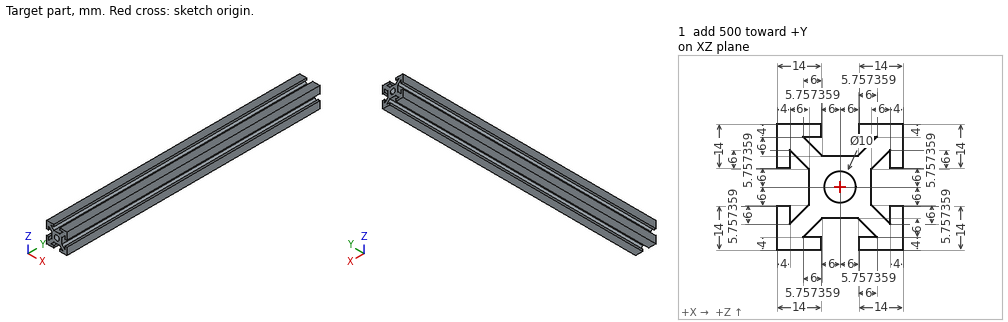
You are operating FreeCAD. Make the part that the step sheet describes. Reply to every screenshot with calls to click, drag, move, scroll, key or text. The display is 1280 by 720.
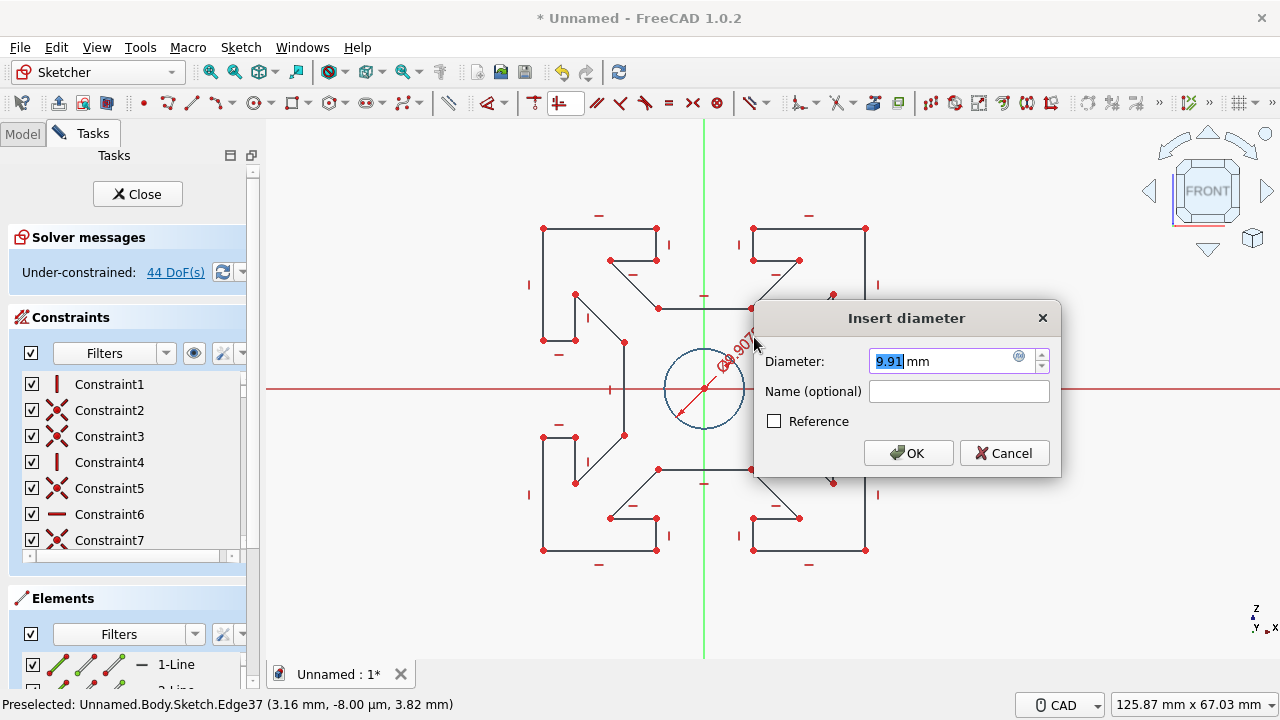
text(10)
key(Return)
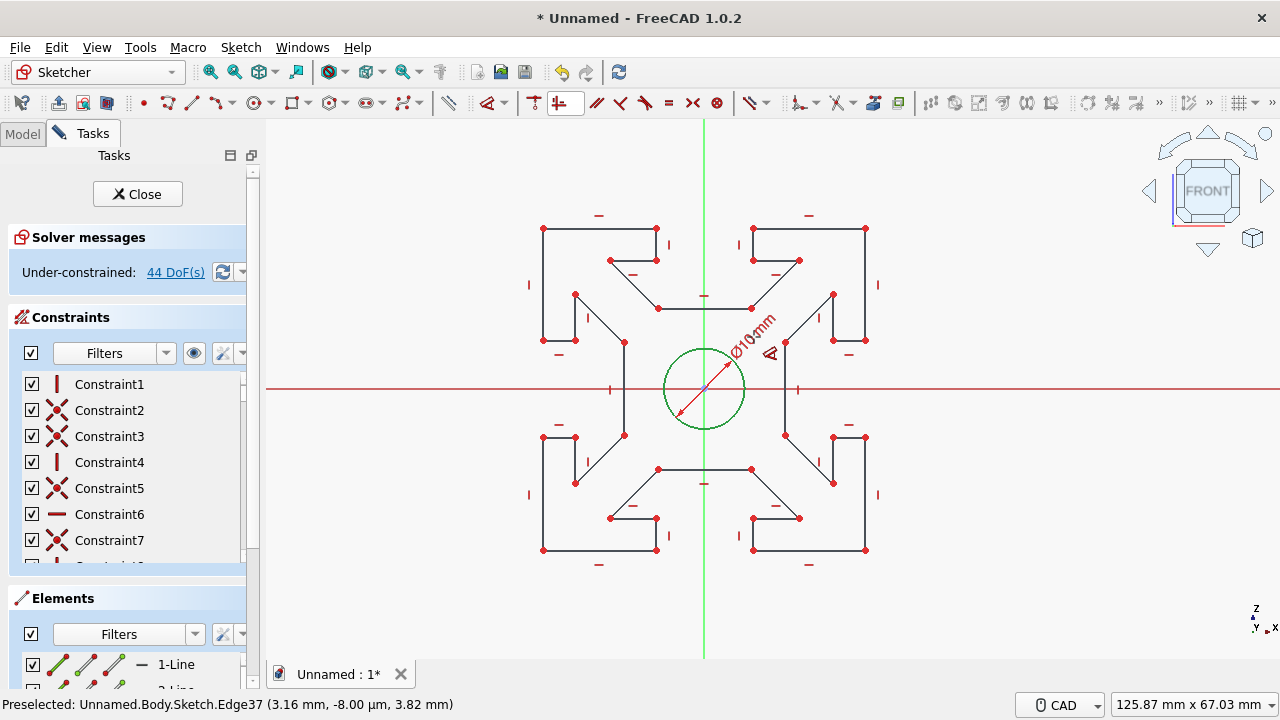
scroll(565, 341, up, 2)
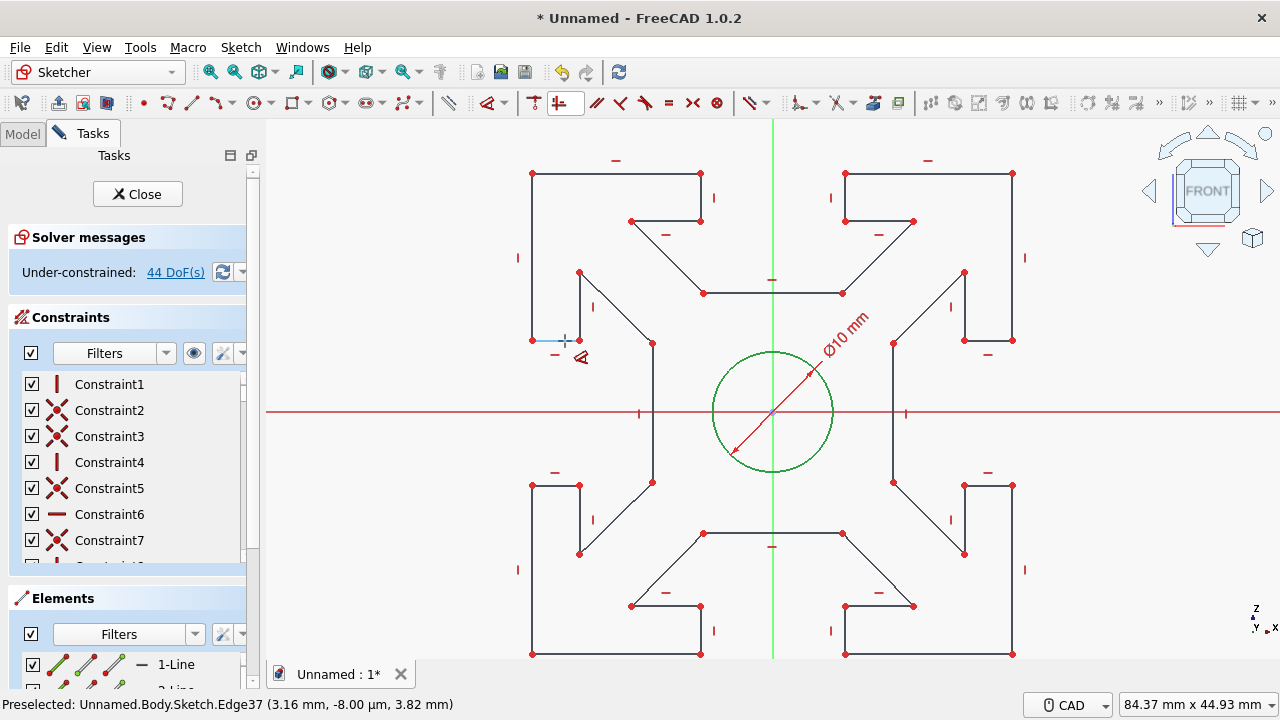
click(565, 341)
click(556, 307)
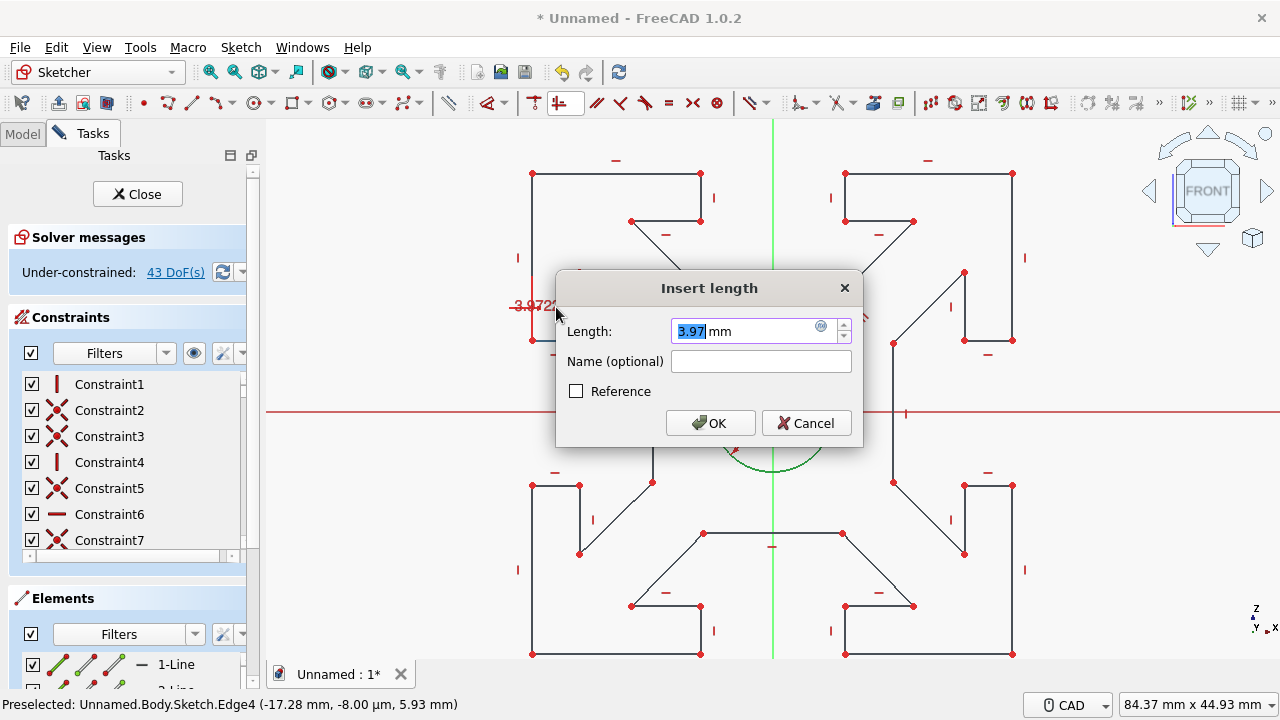
text(4)
key(Return)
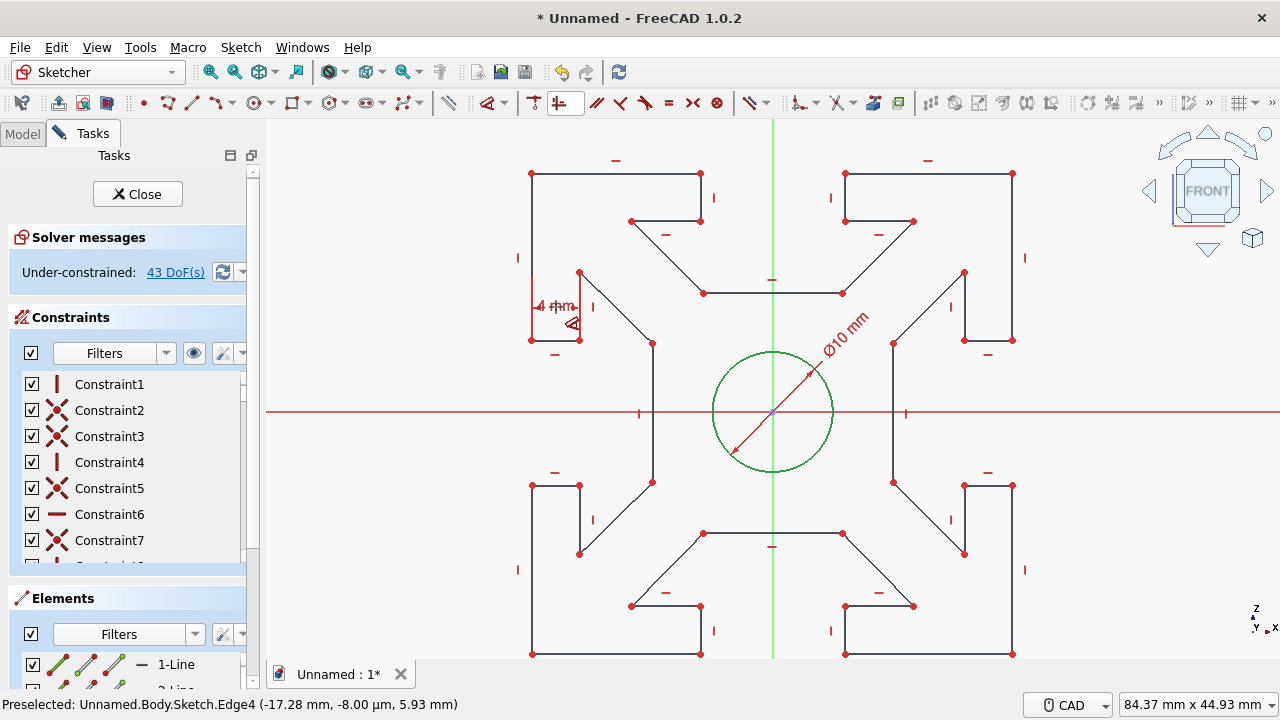
click(701, 188)
click(667, 198)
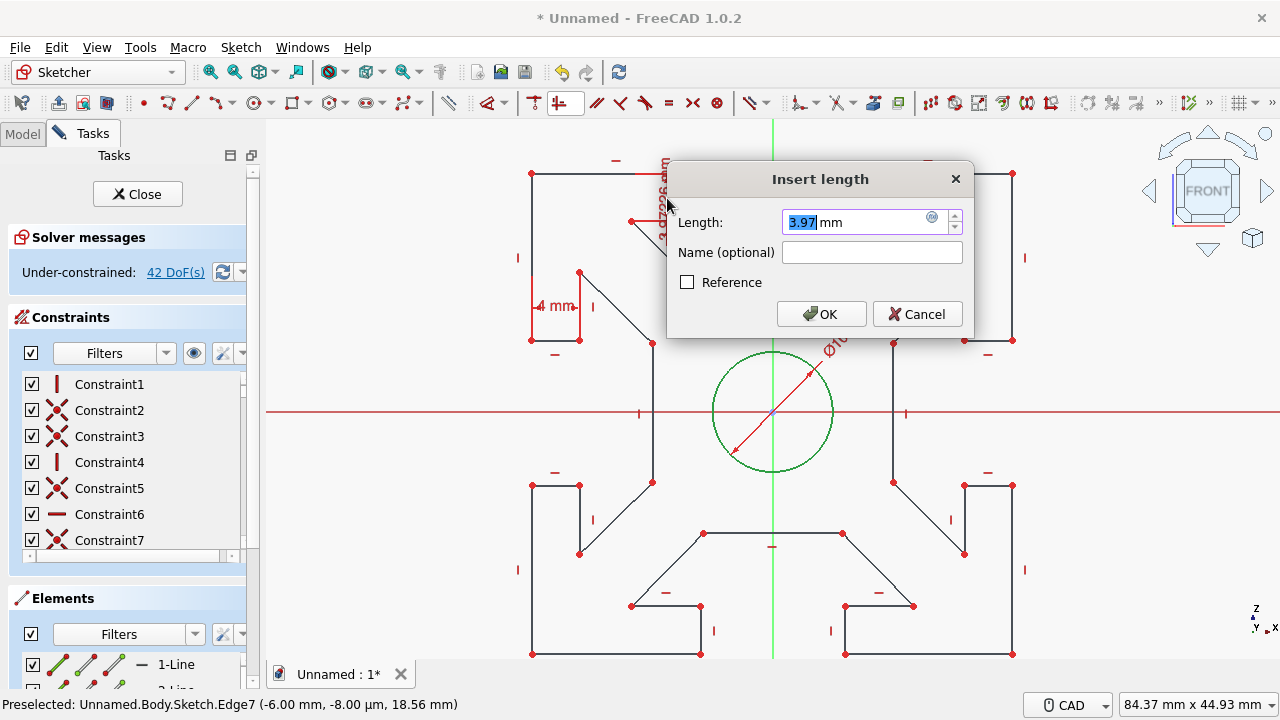
text(4)
key(Return)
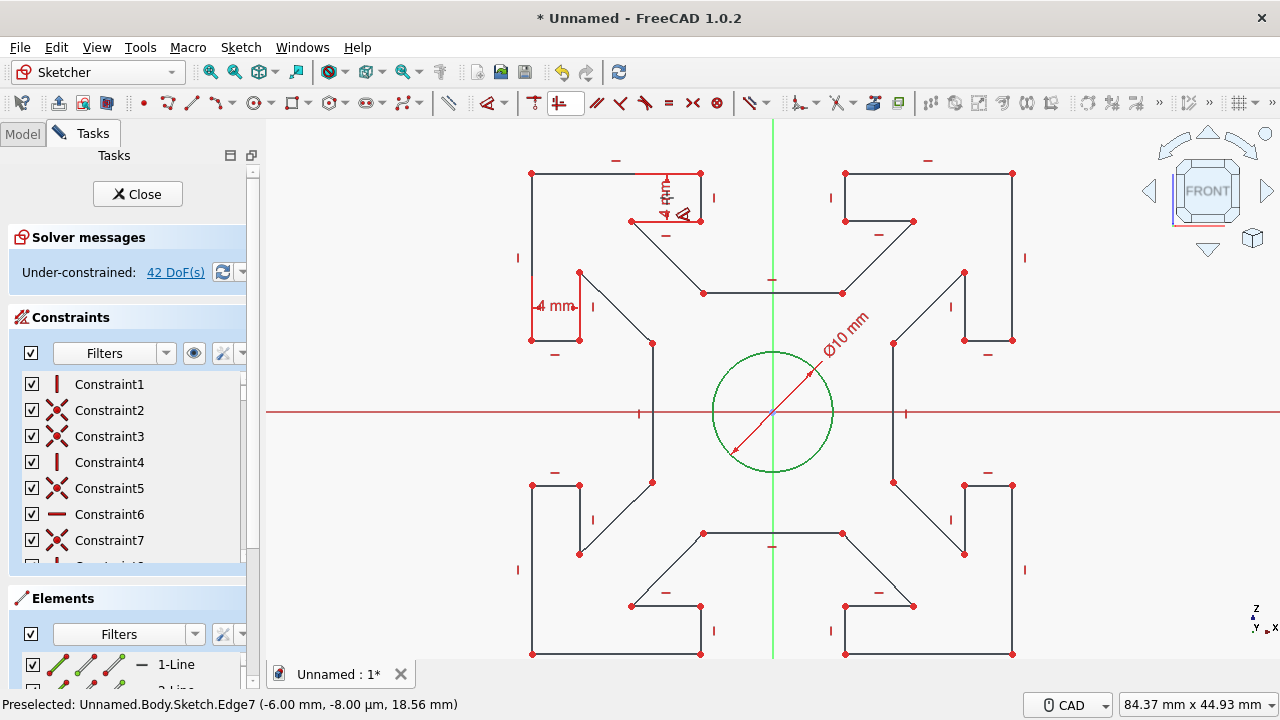
click(845, 207)
click(879, 198)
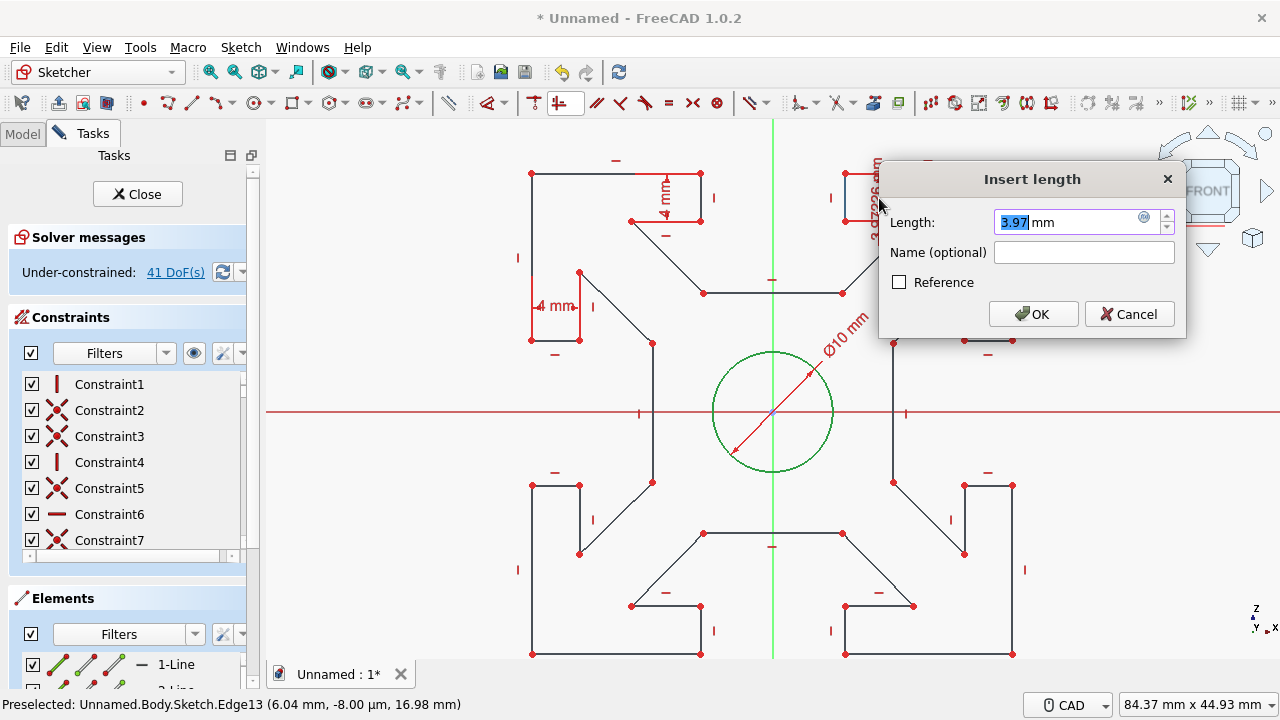
text(4)
key(Return)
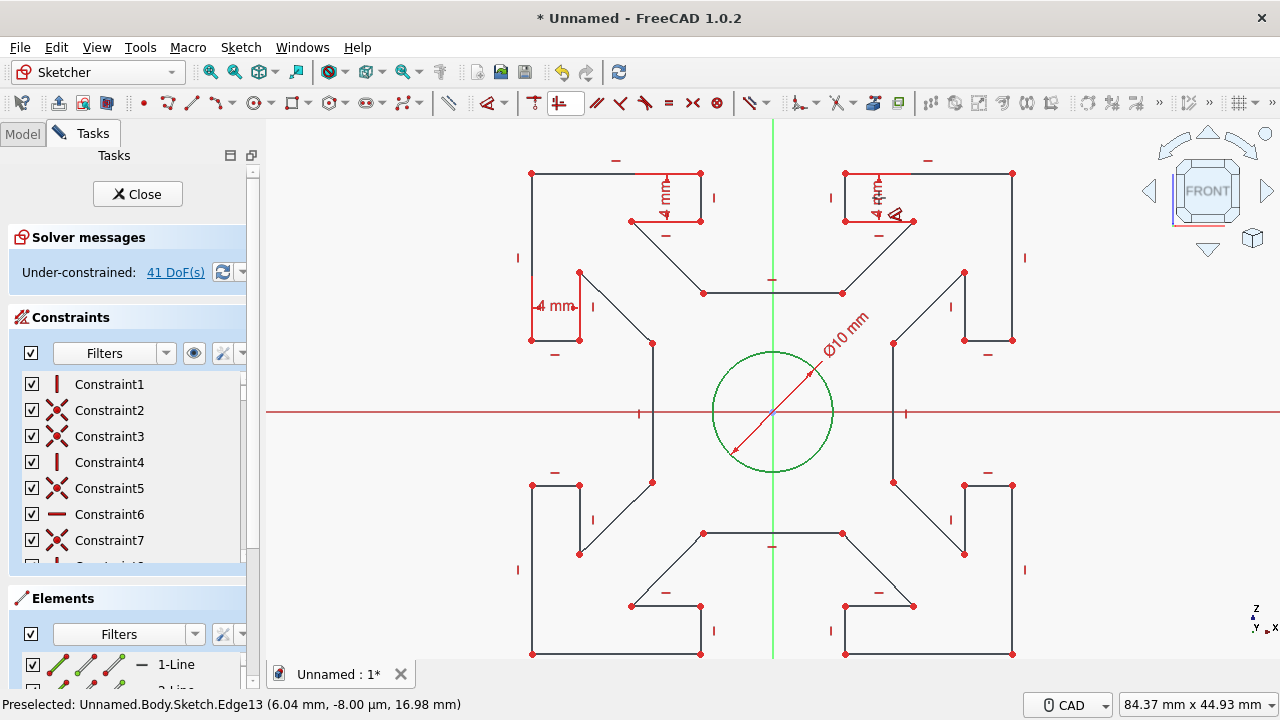
click(998, 341)
click(989, 307)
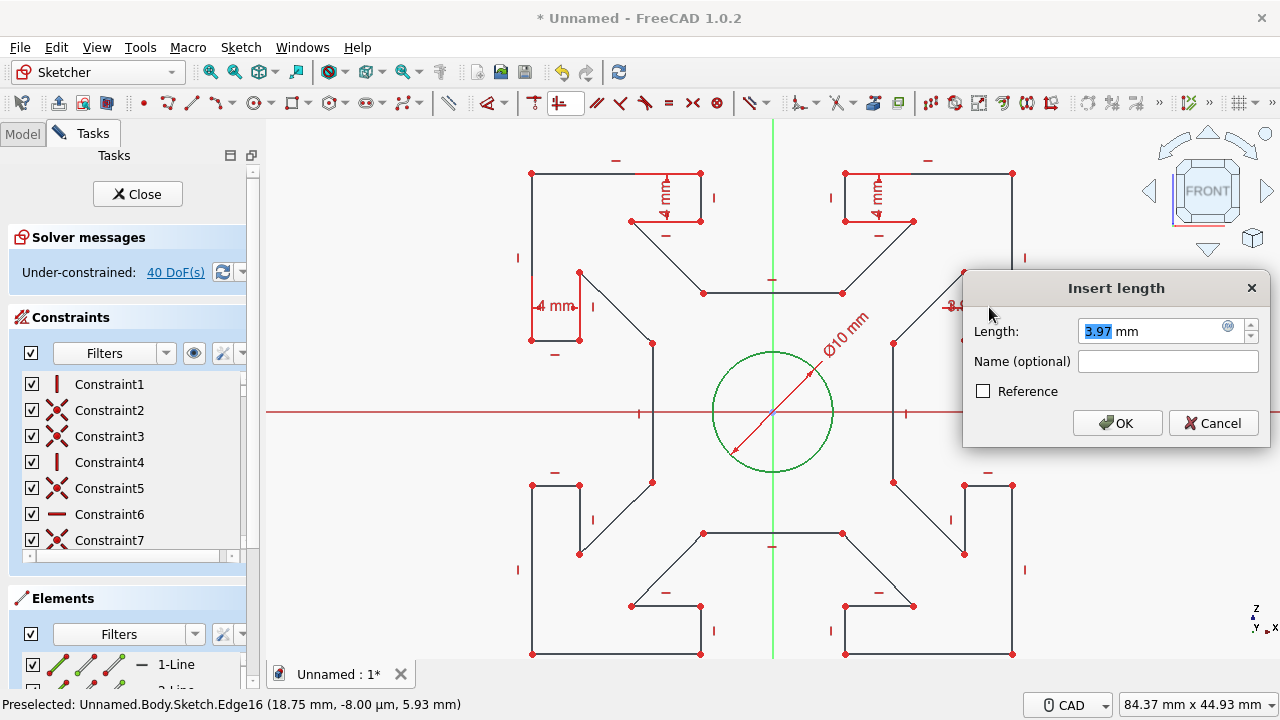
text(4)
key(Return)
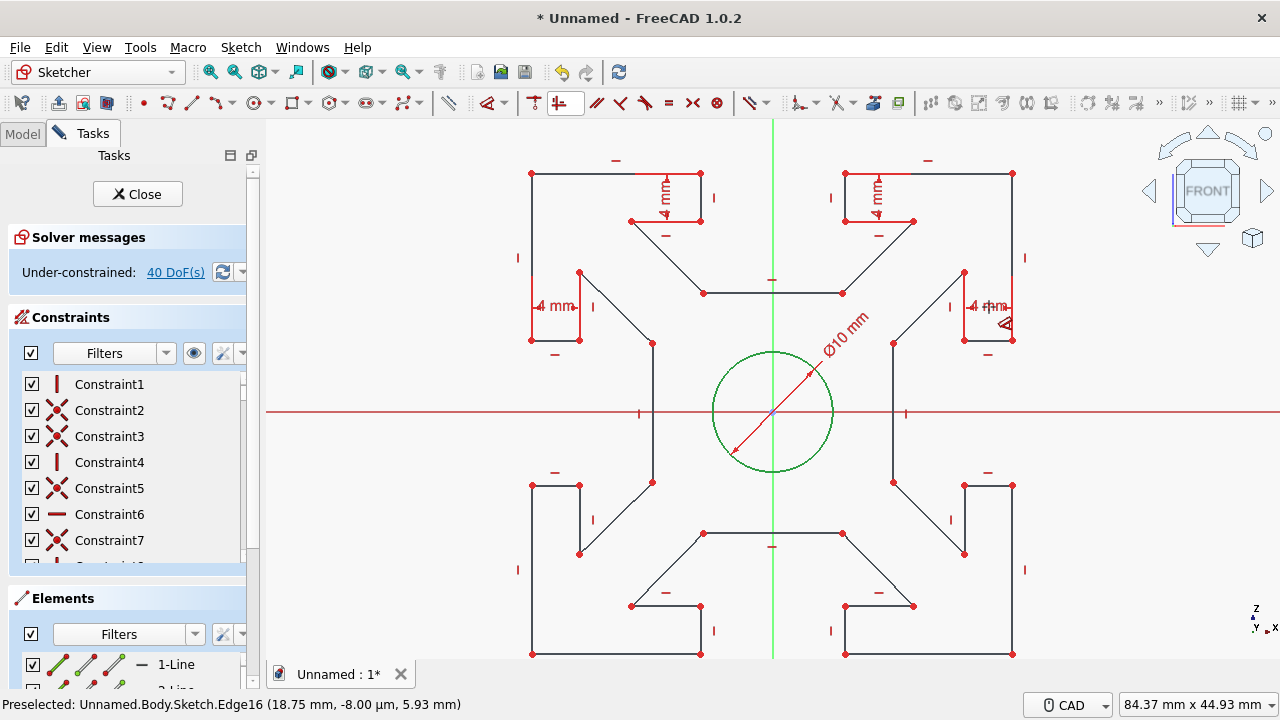
click(979, 486)
click(989, 520)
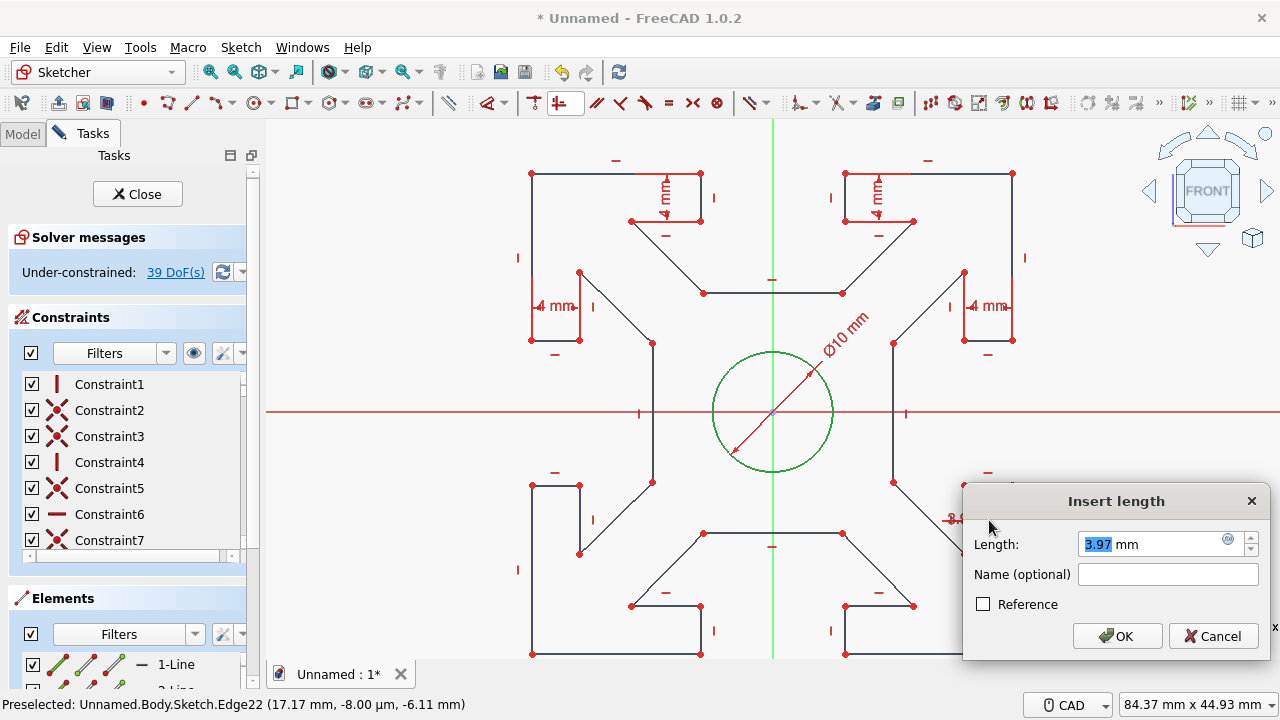
text(4)
key(Return)